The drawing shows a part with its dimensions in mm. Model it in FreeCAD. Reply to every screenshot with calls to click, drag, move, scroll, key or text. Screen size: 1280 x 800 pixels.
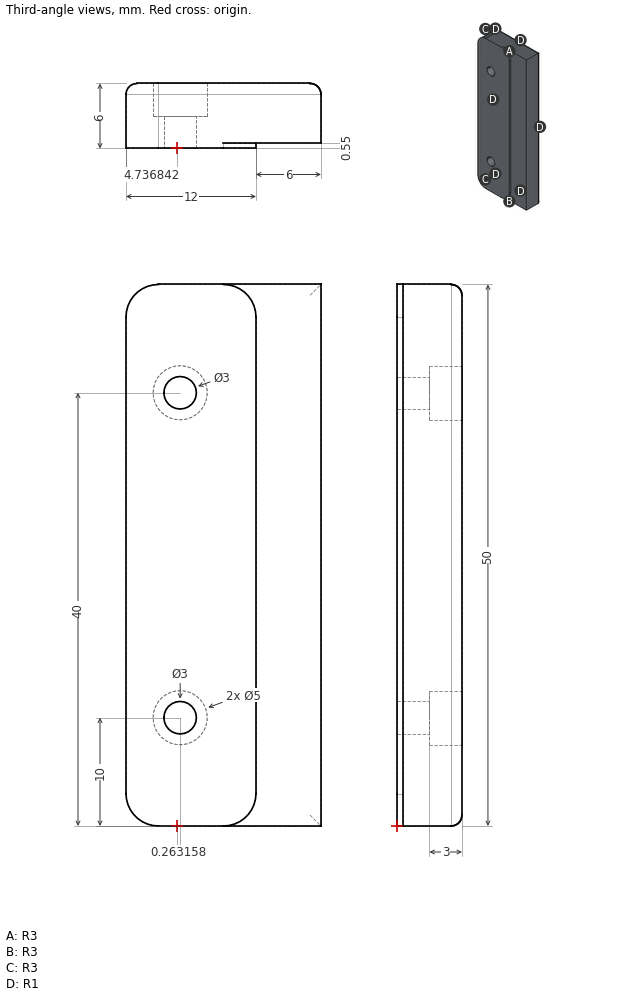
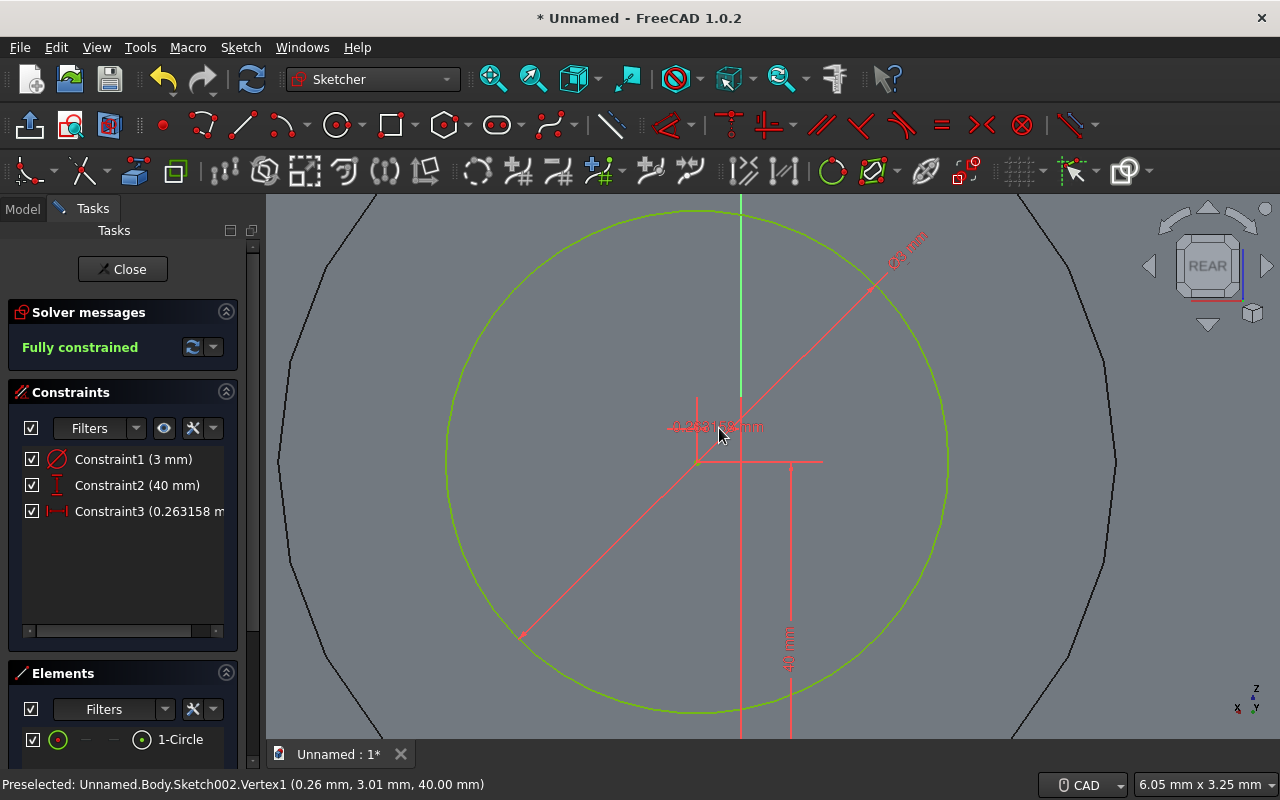
click(123, 269)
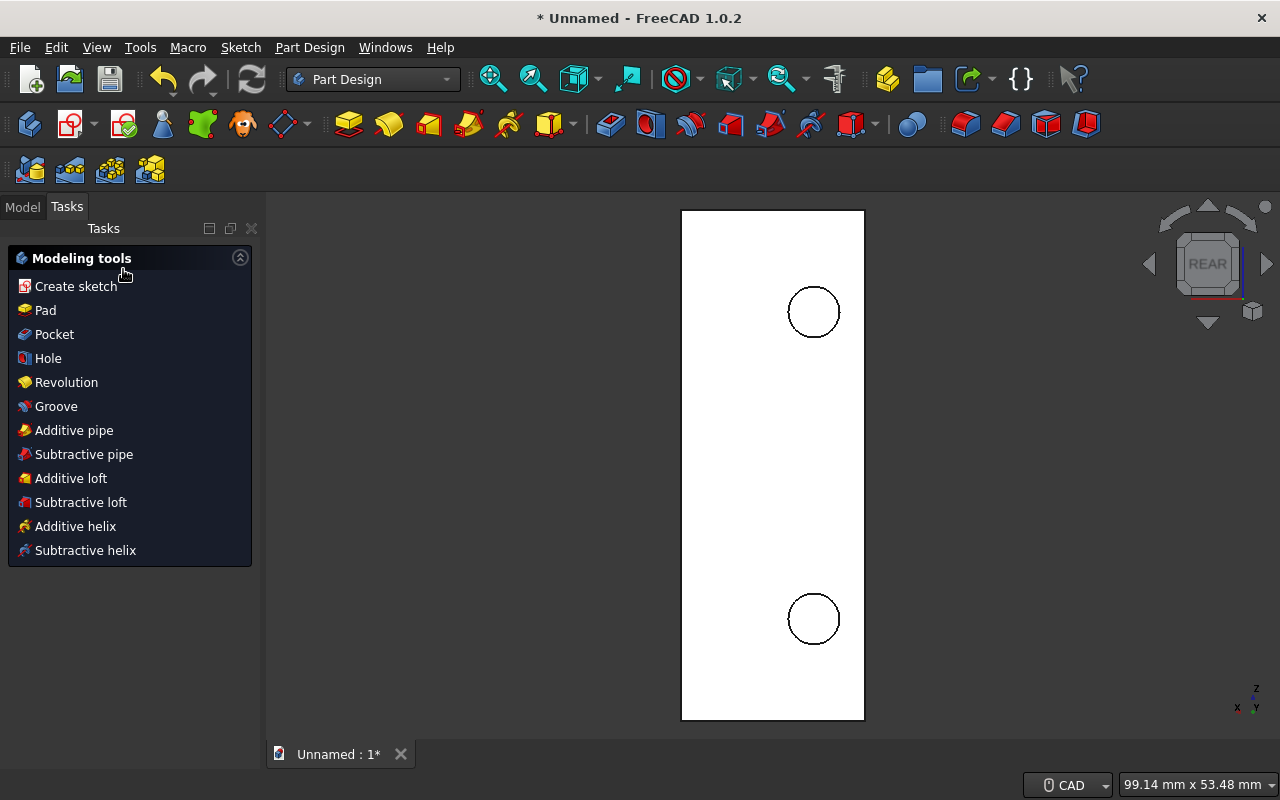
click(612, 124)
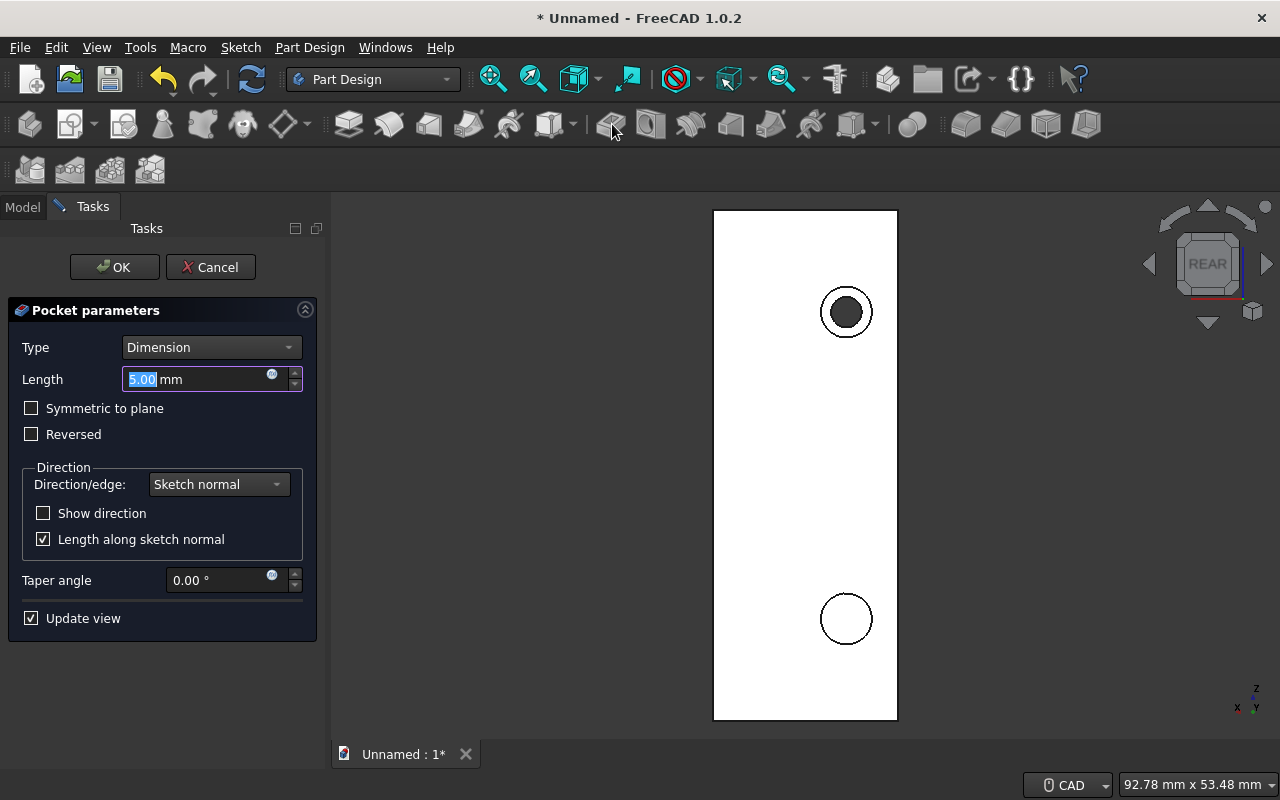
click(212, 348)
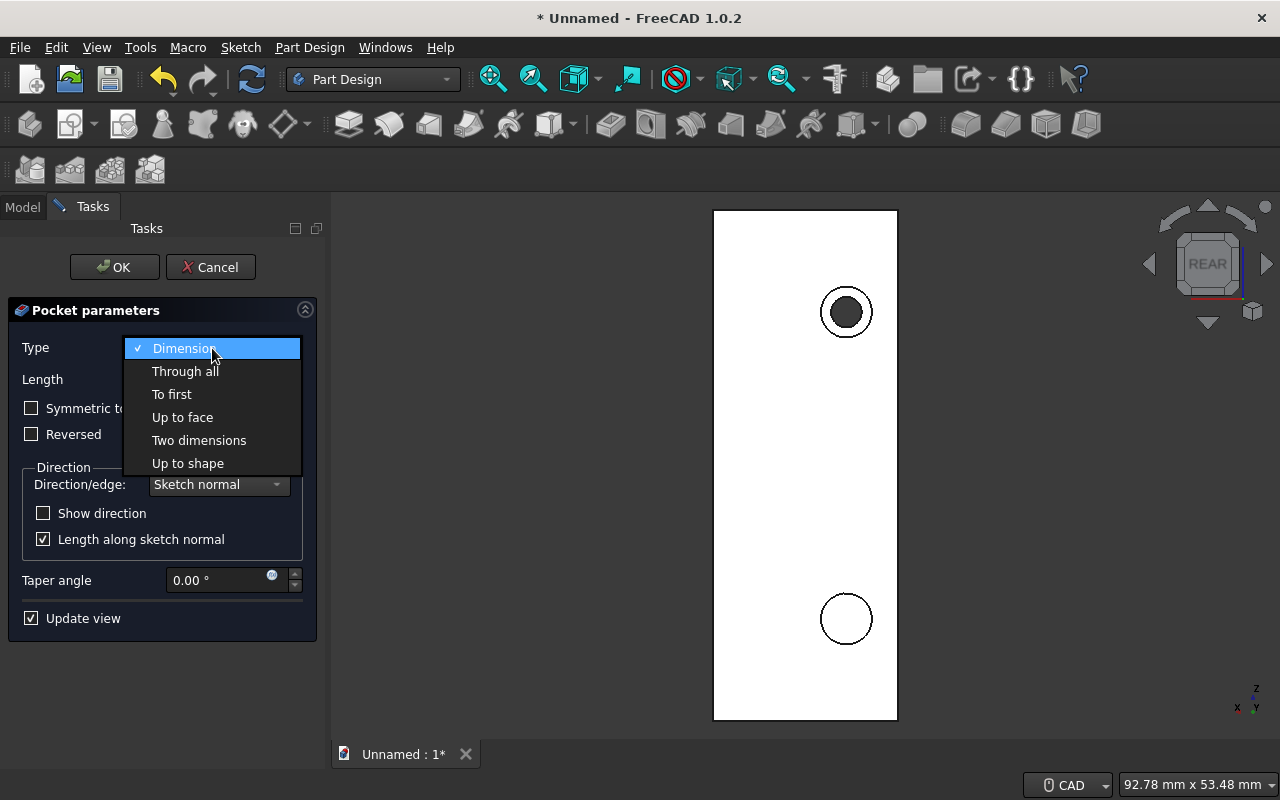
click(212, 372)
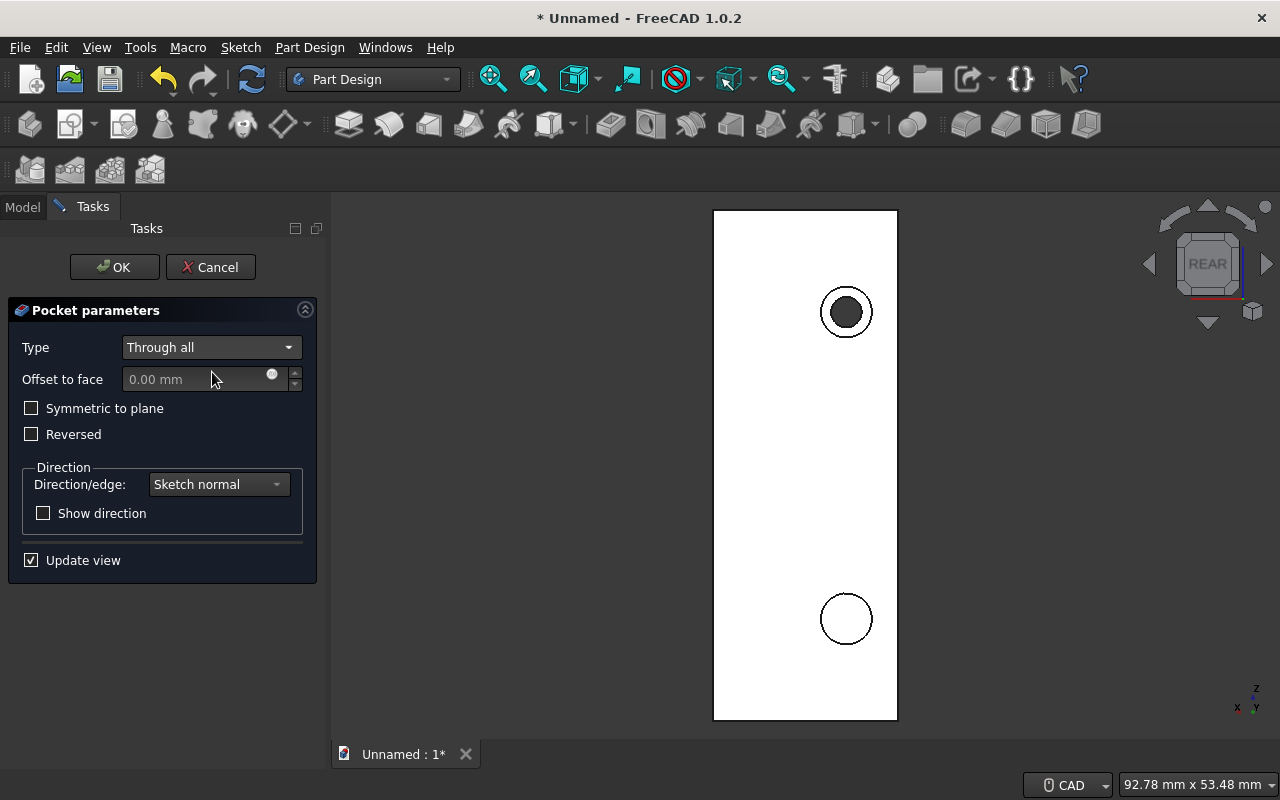
click(115, 267)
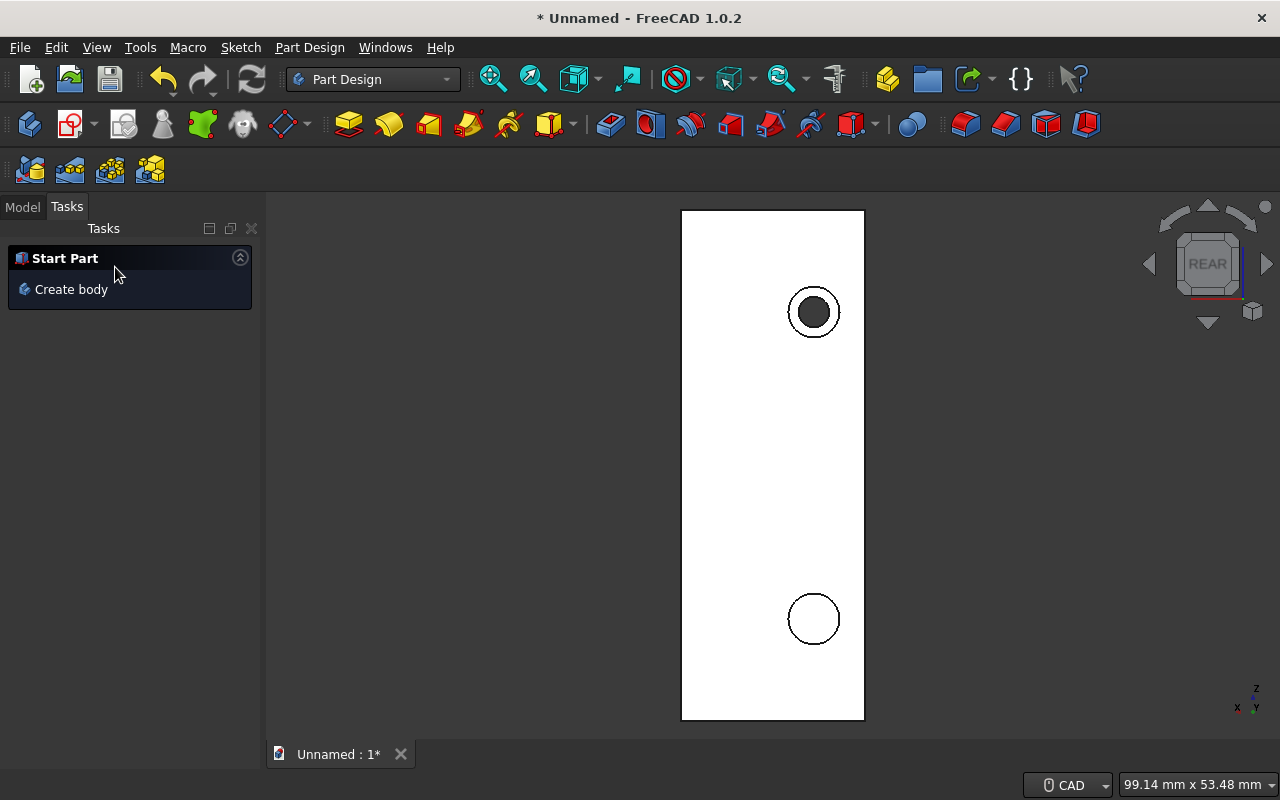
click(814, 618)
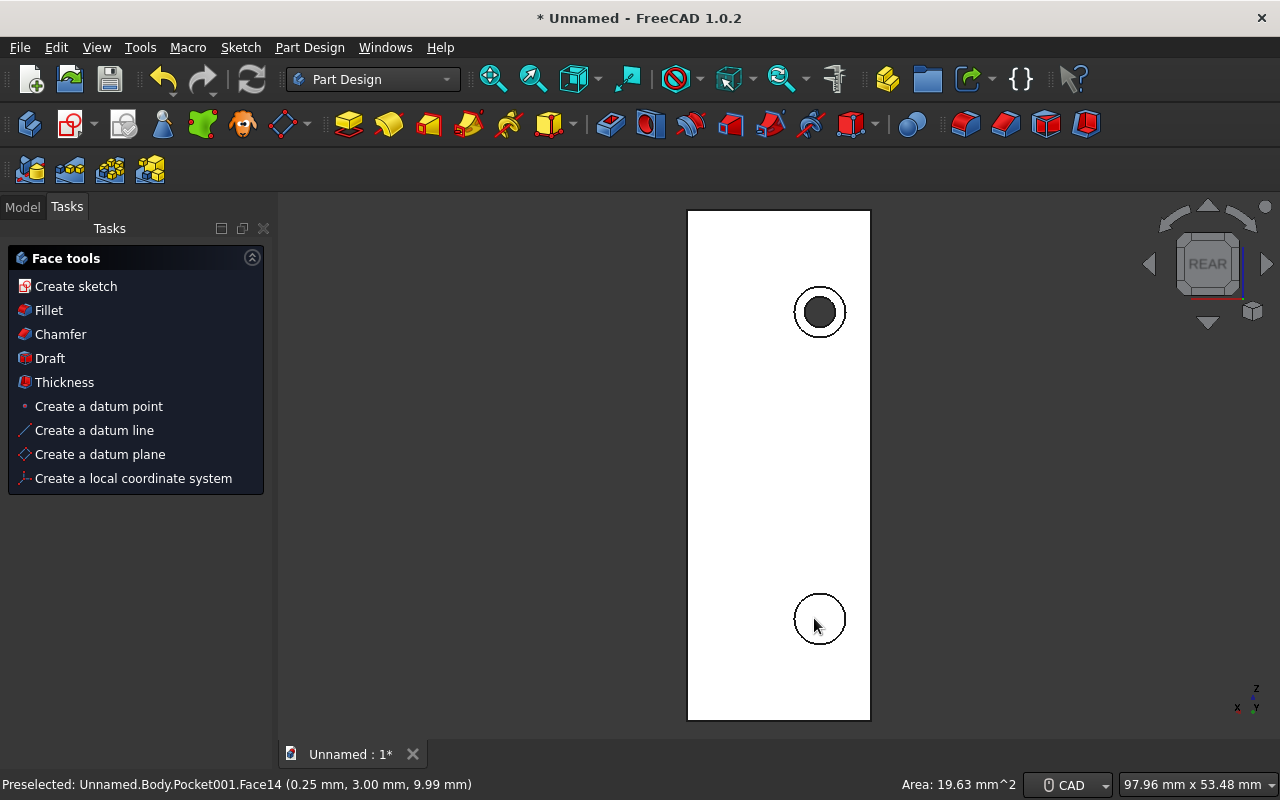
click(70, 124)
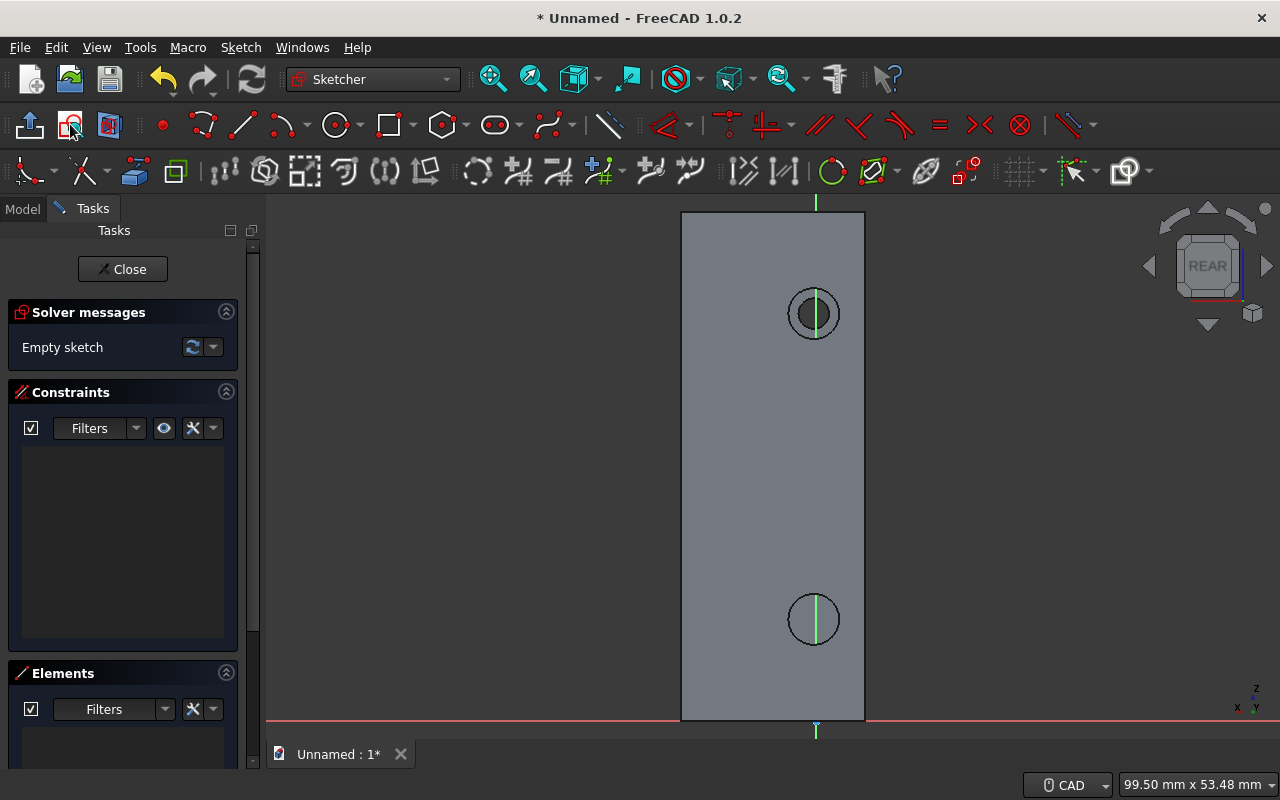
scroll(825, 635, up, 12)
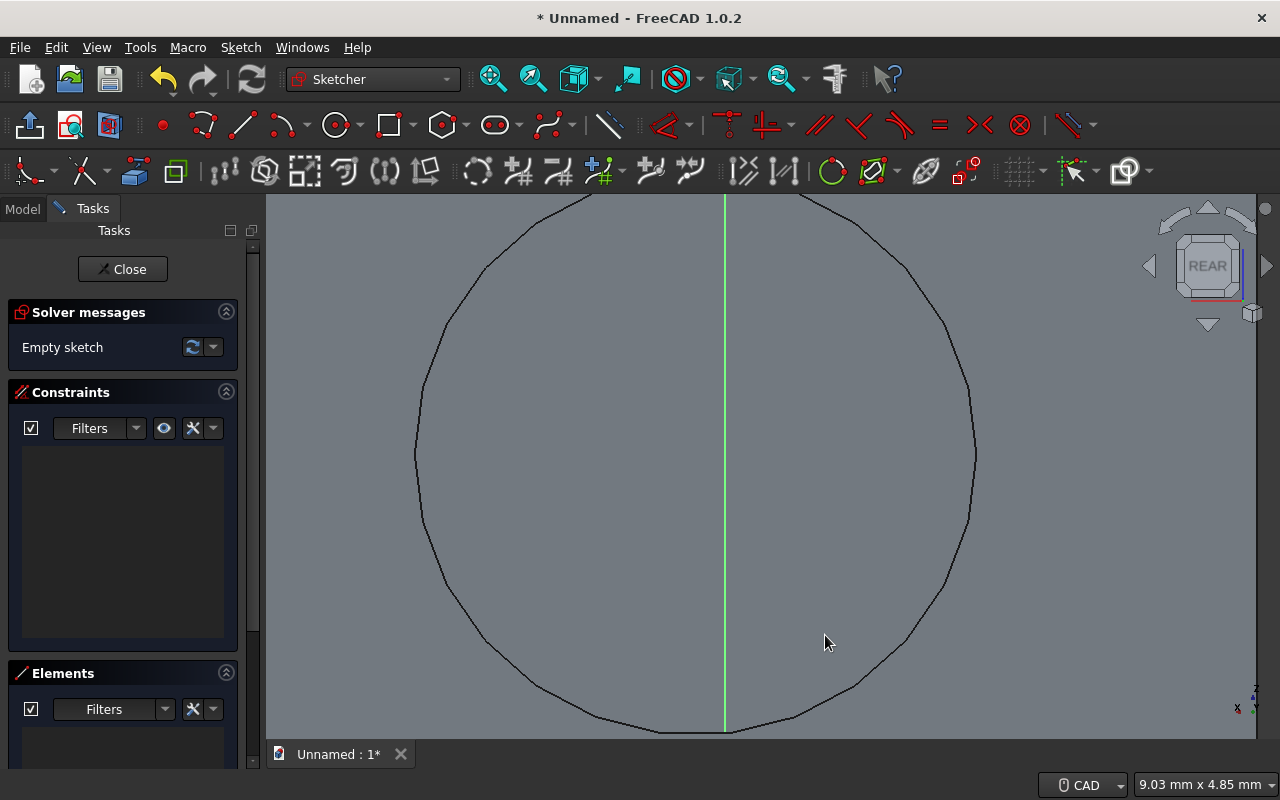
click(336, 126)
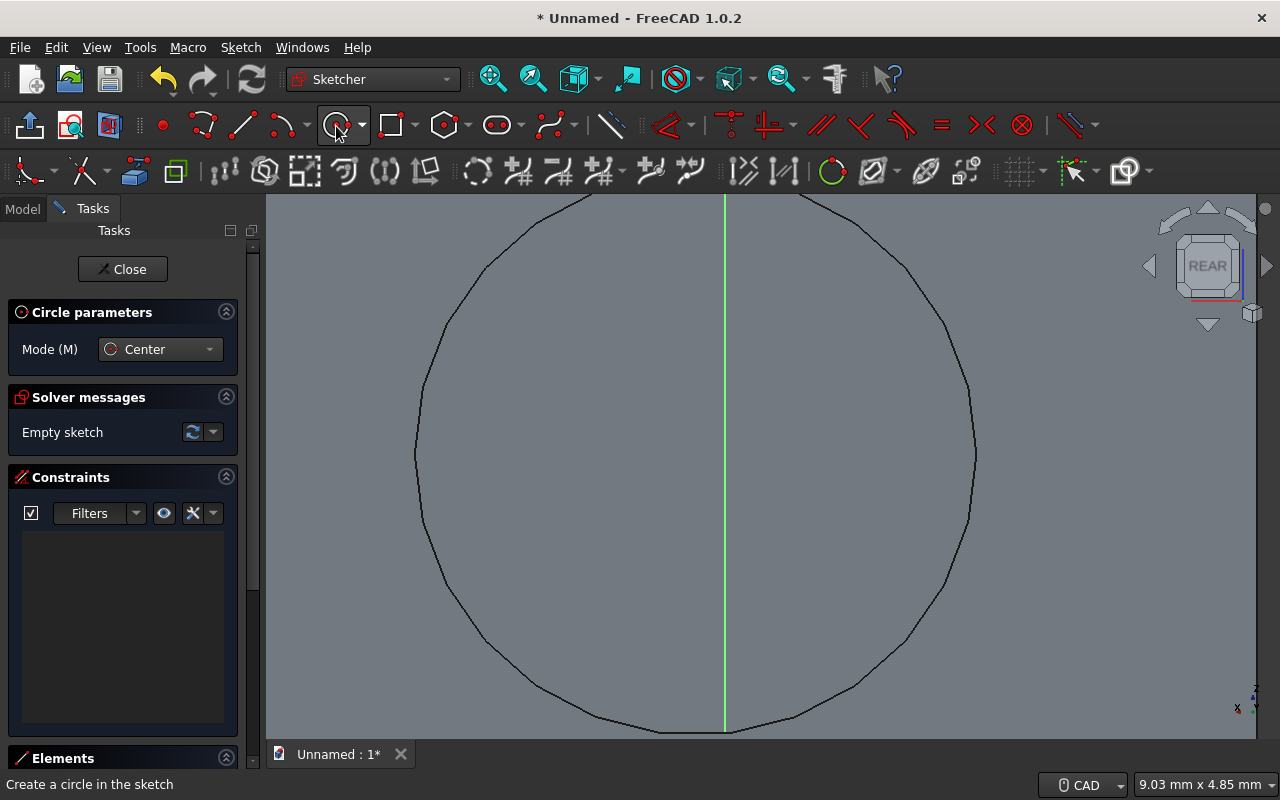
click(696, 455)
click(815, 335)
key(Escape)